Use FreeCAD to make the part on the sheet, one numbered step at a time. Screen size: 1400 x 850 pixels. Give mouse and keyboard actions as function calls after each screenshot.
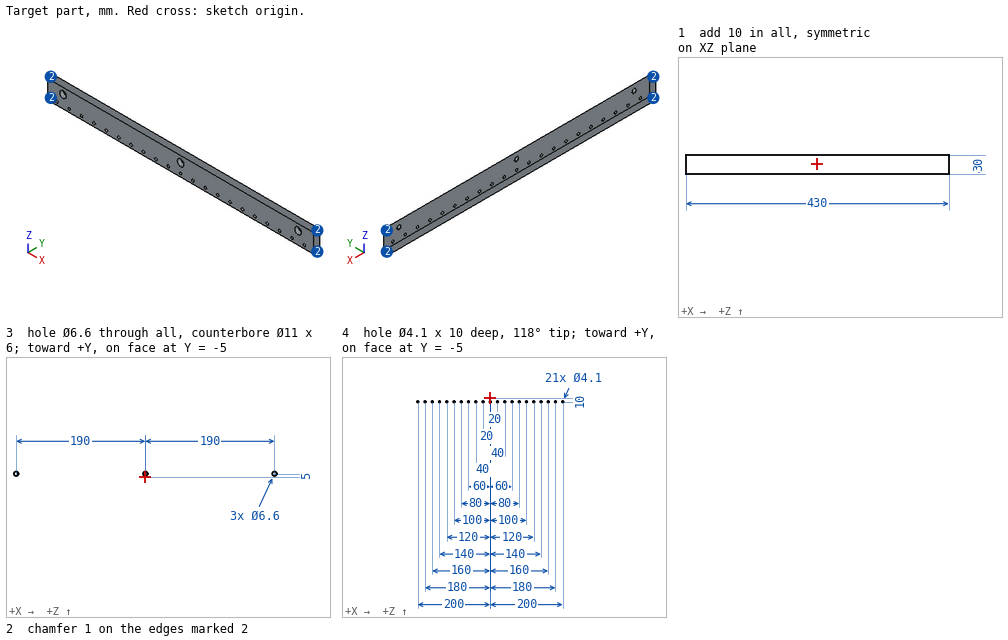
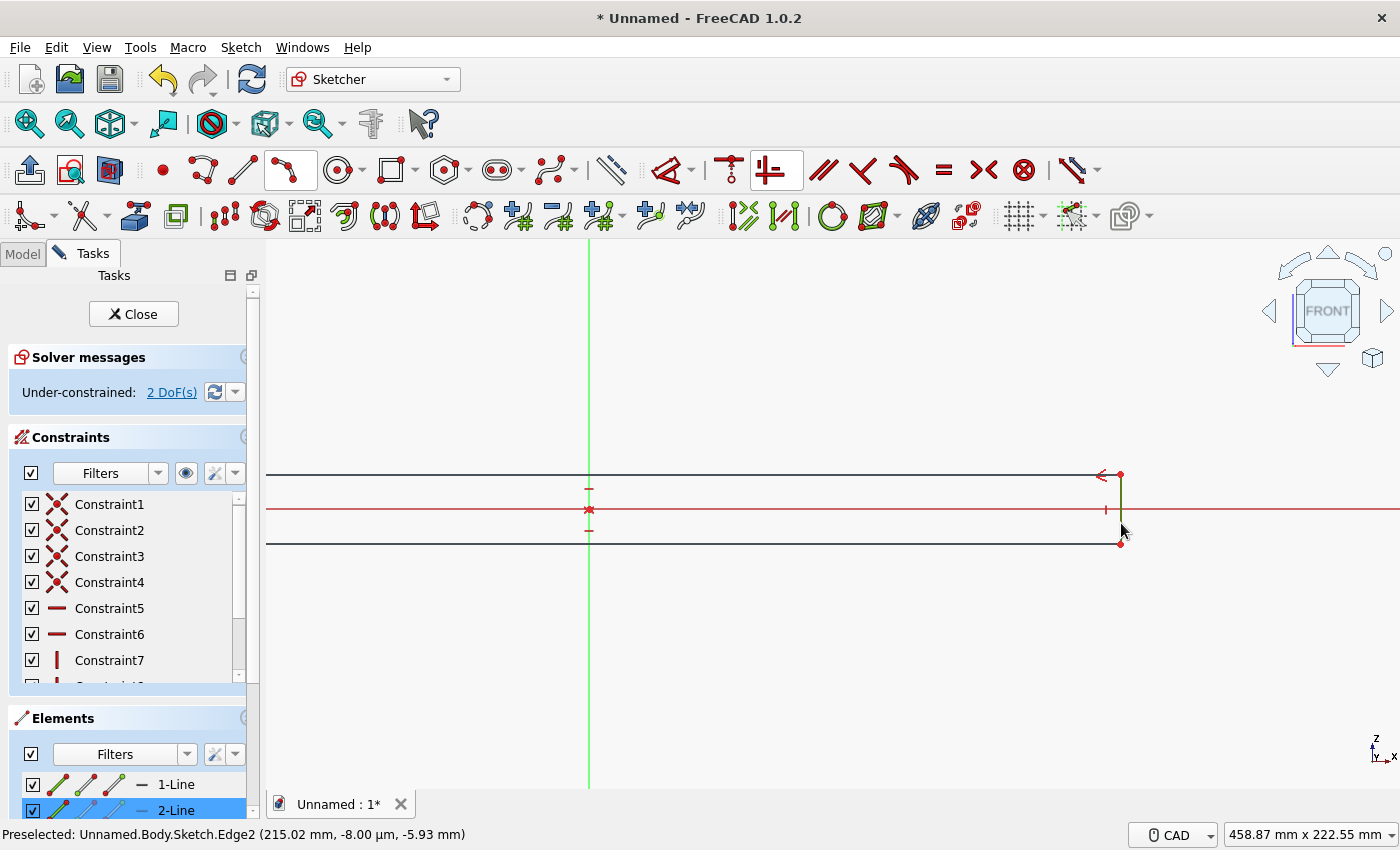
click(694, 170)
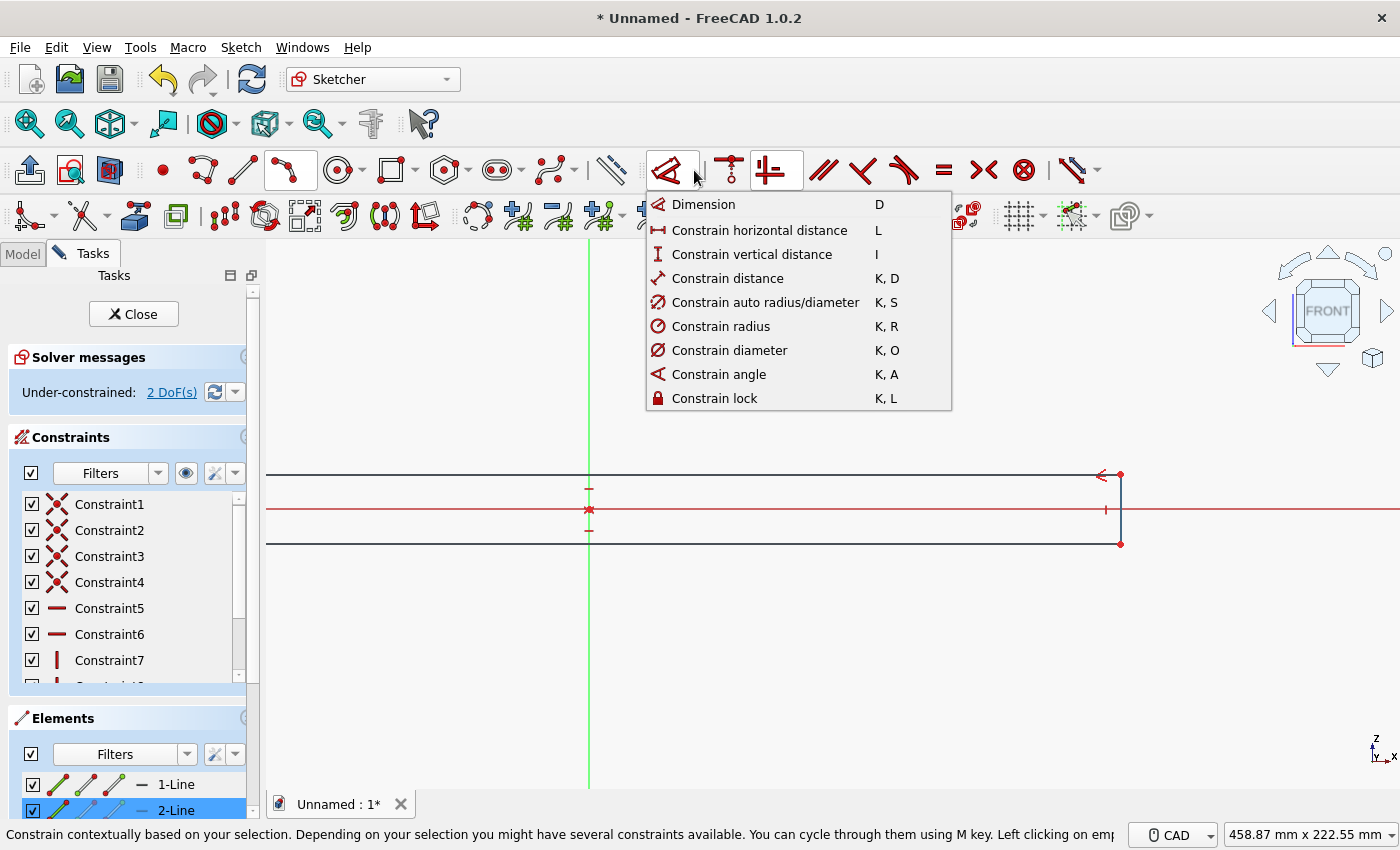
click(799, 254)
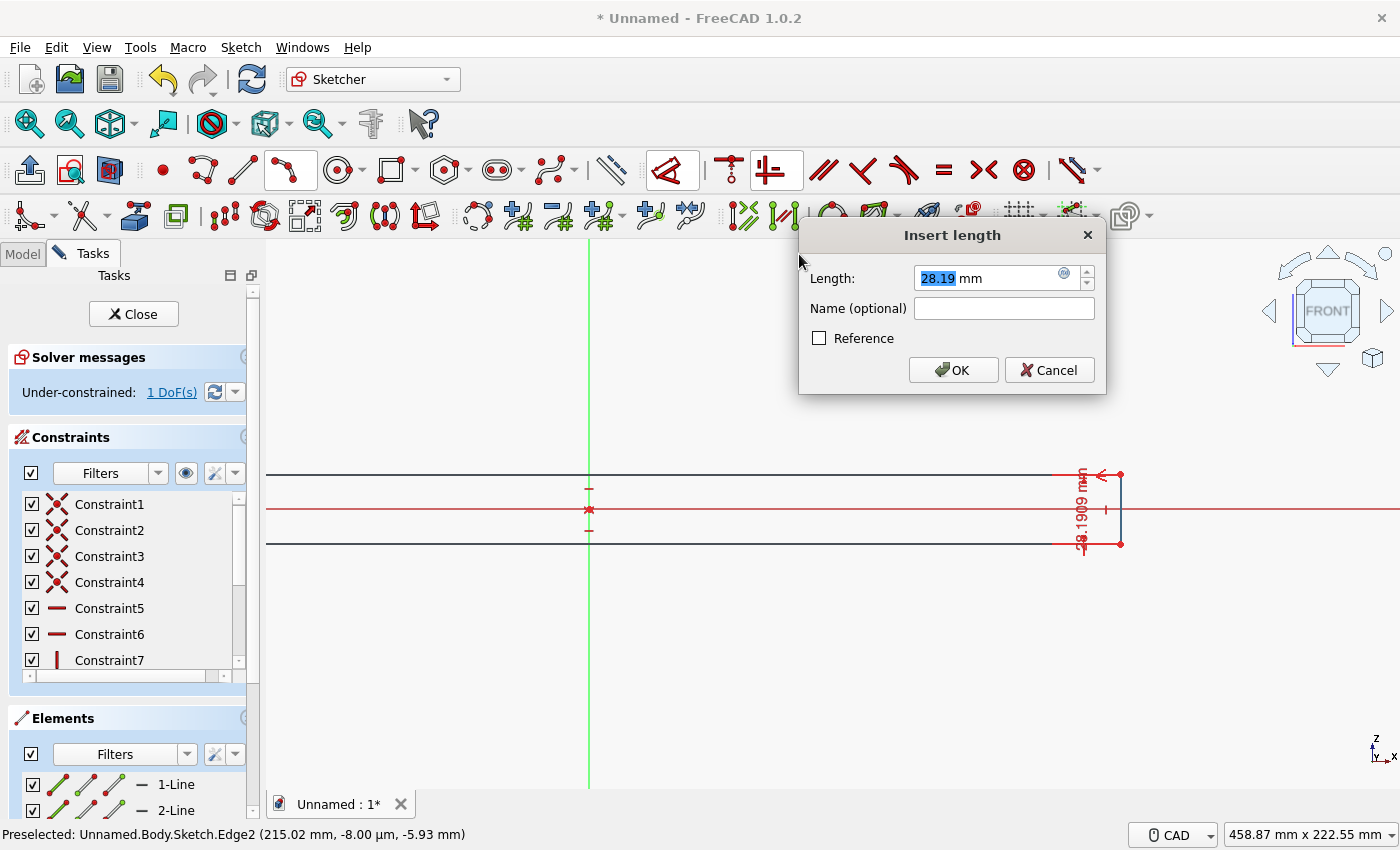
text(30)
key(Return)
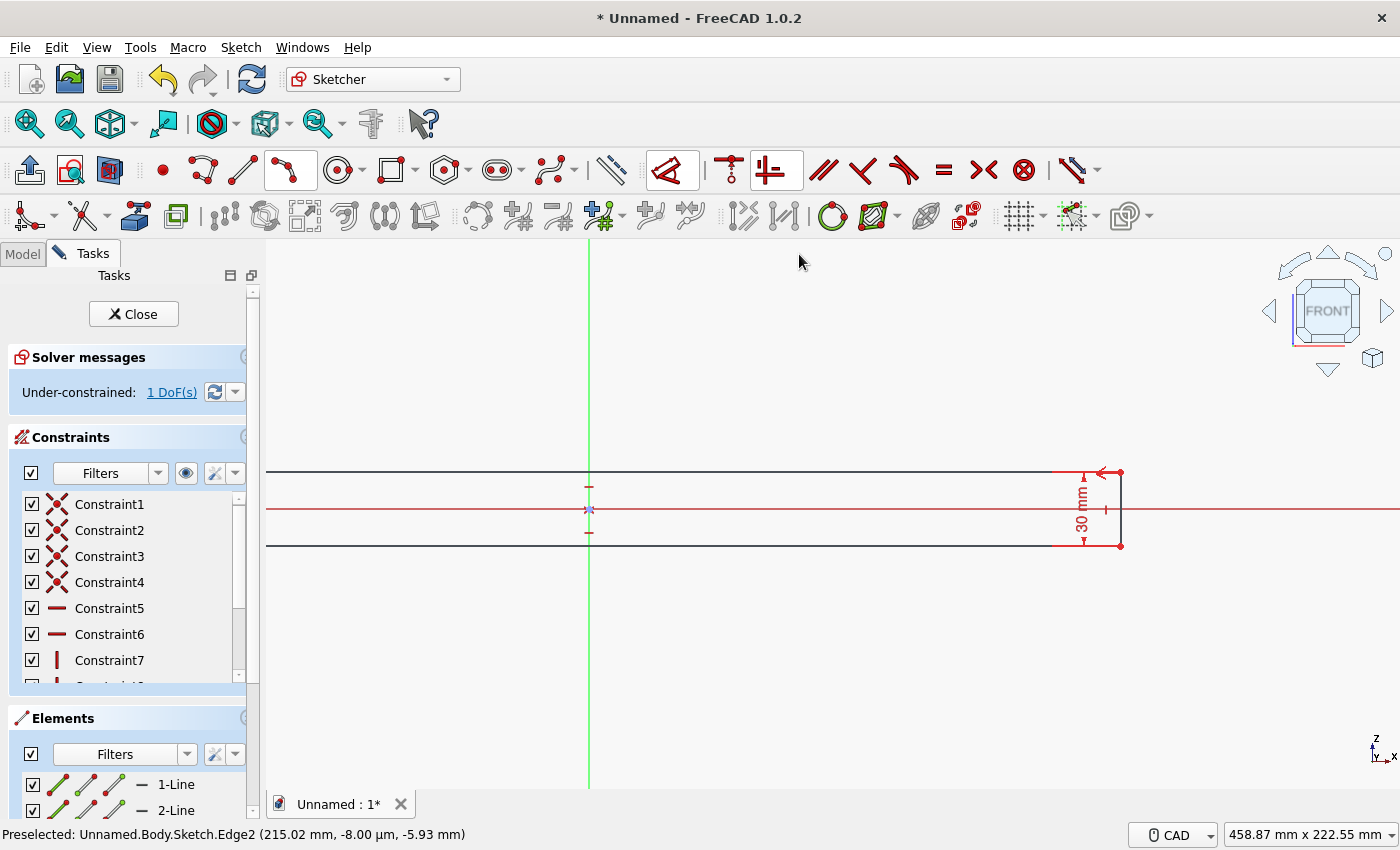
click(377, 546)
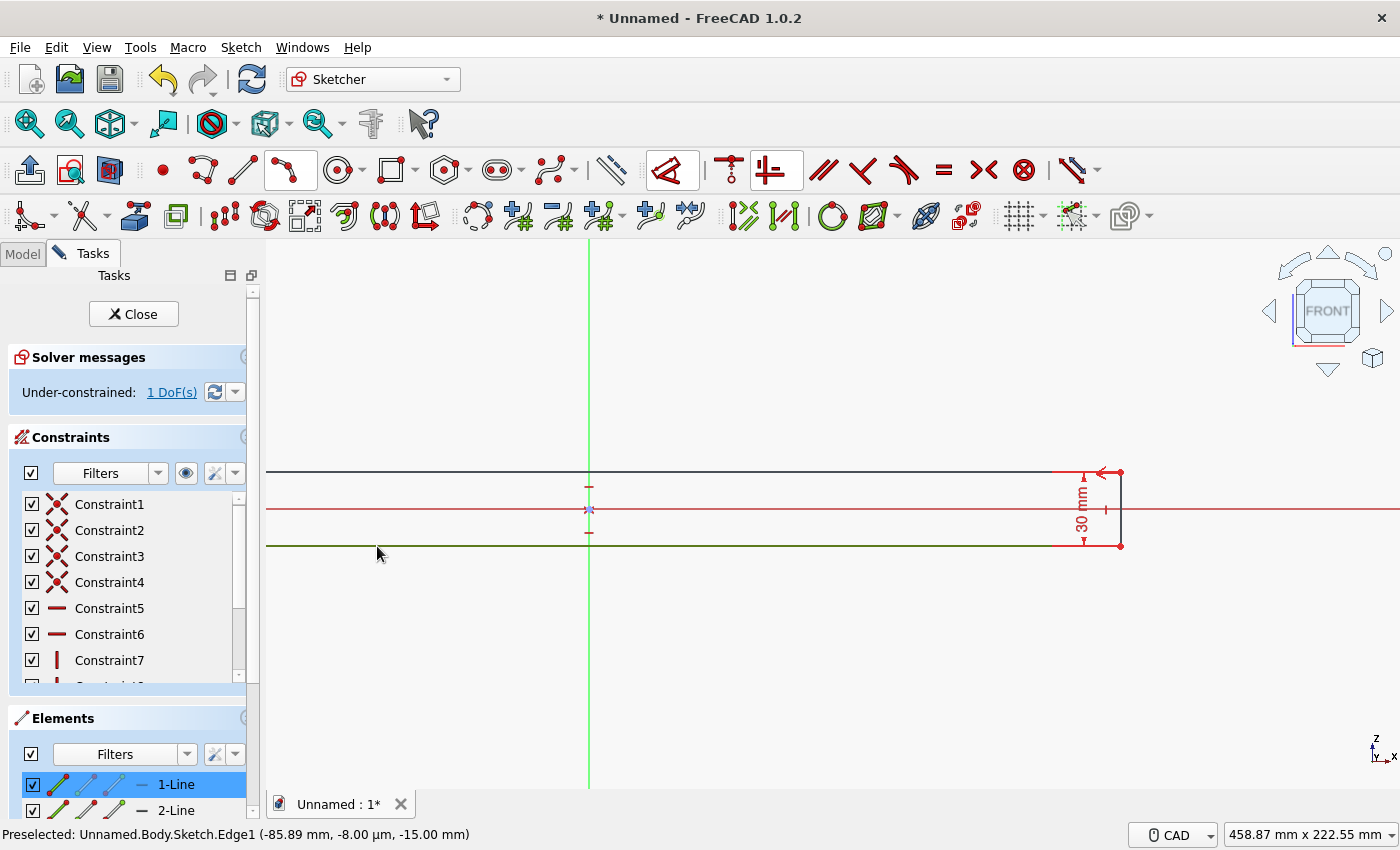
click(694, 170)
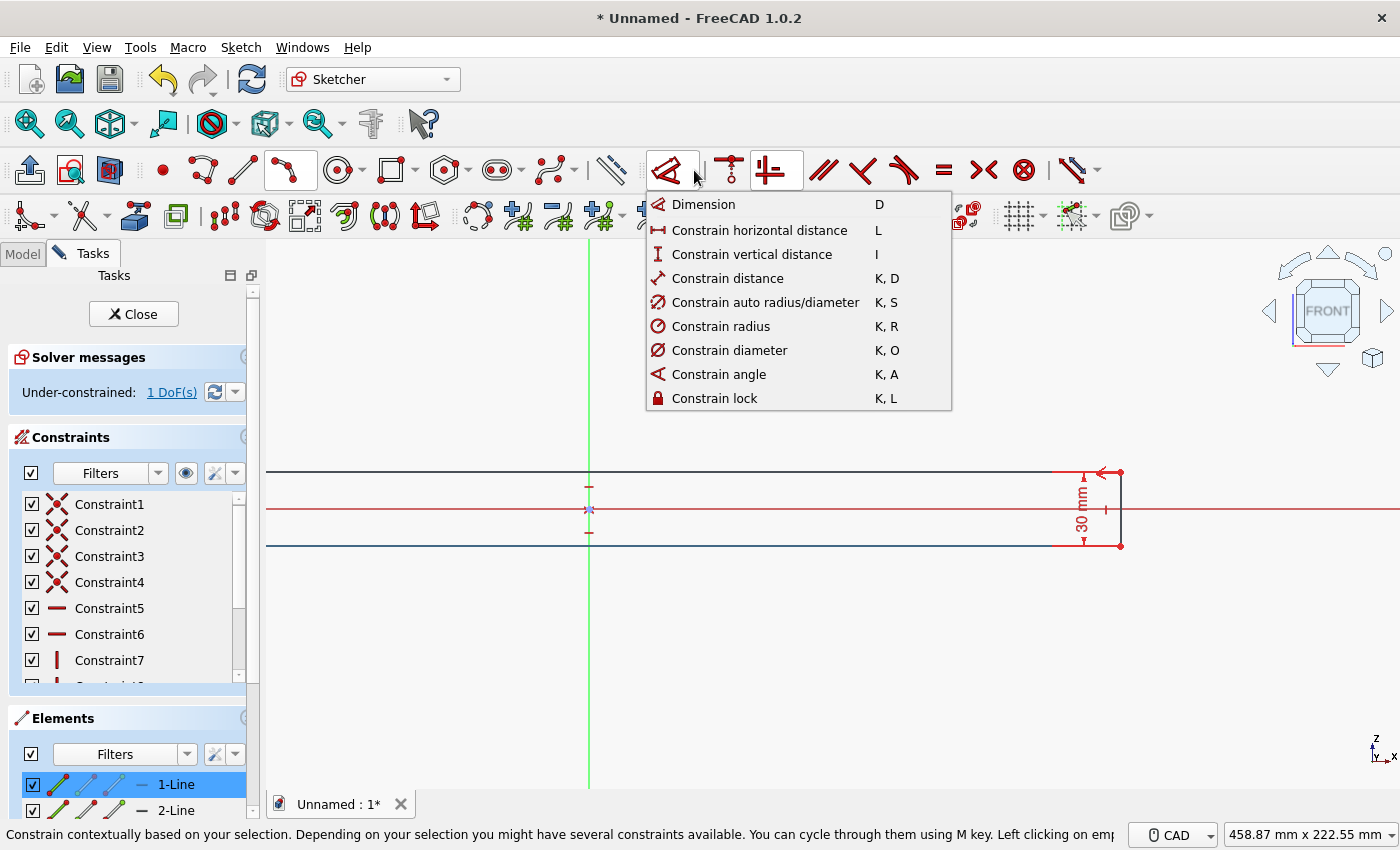
click(799, 230)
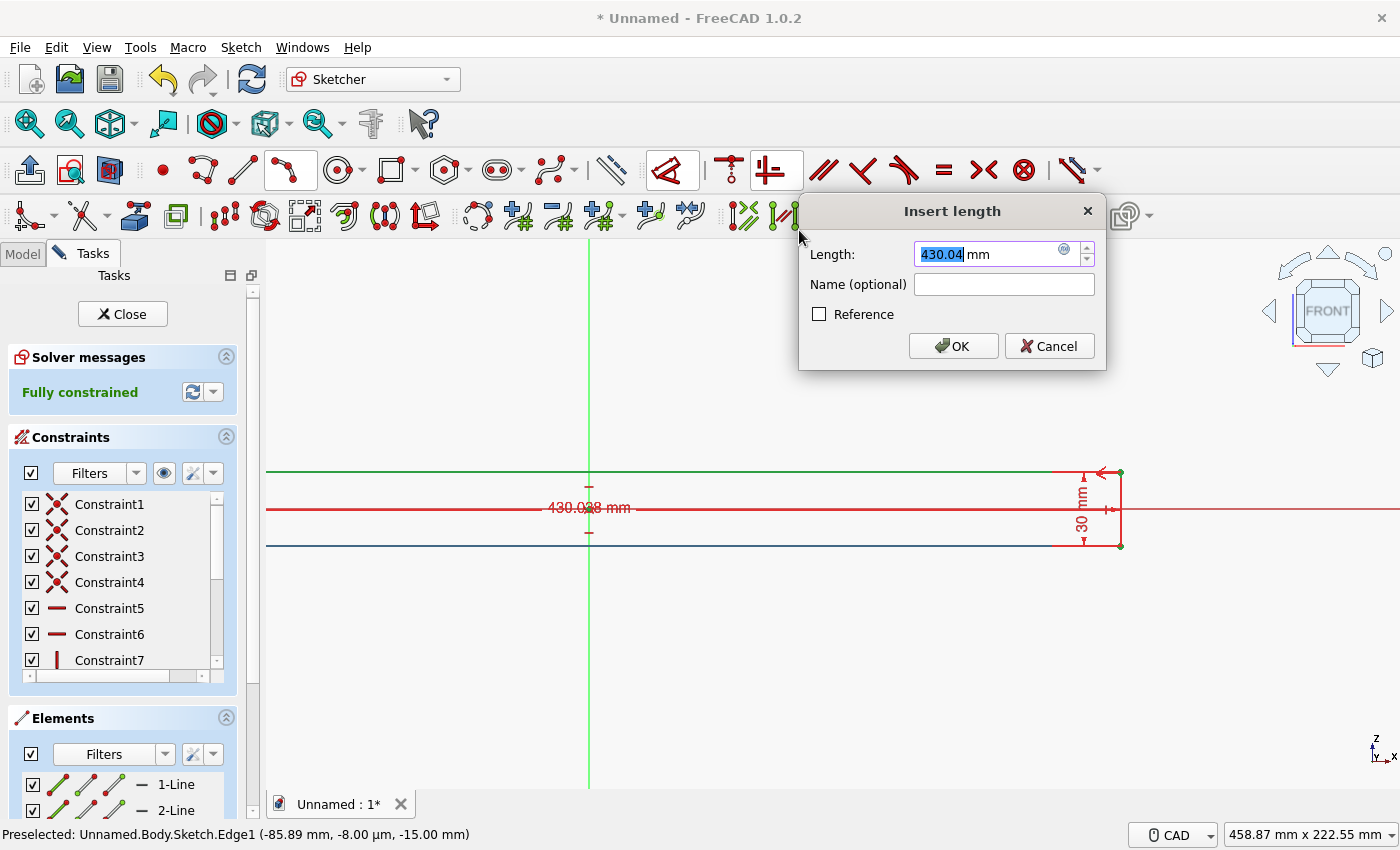
text(430)
key(Return)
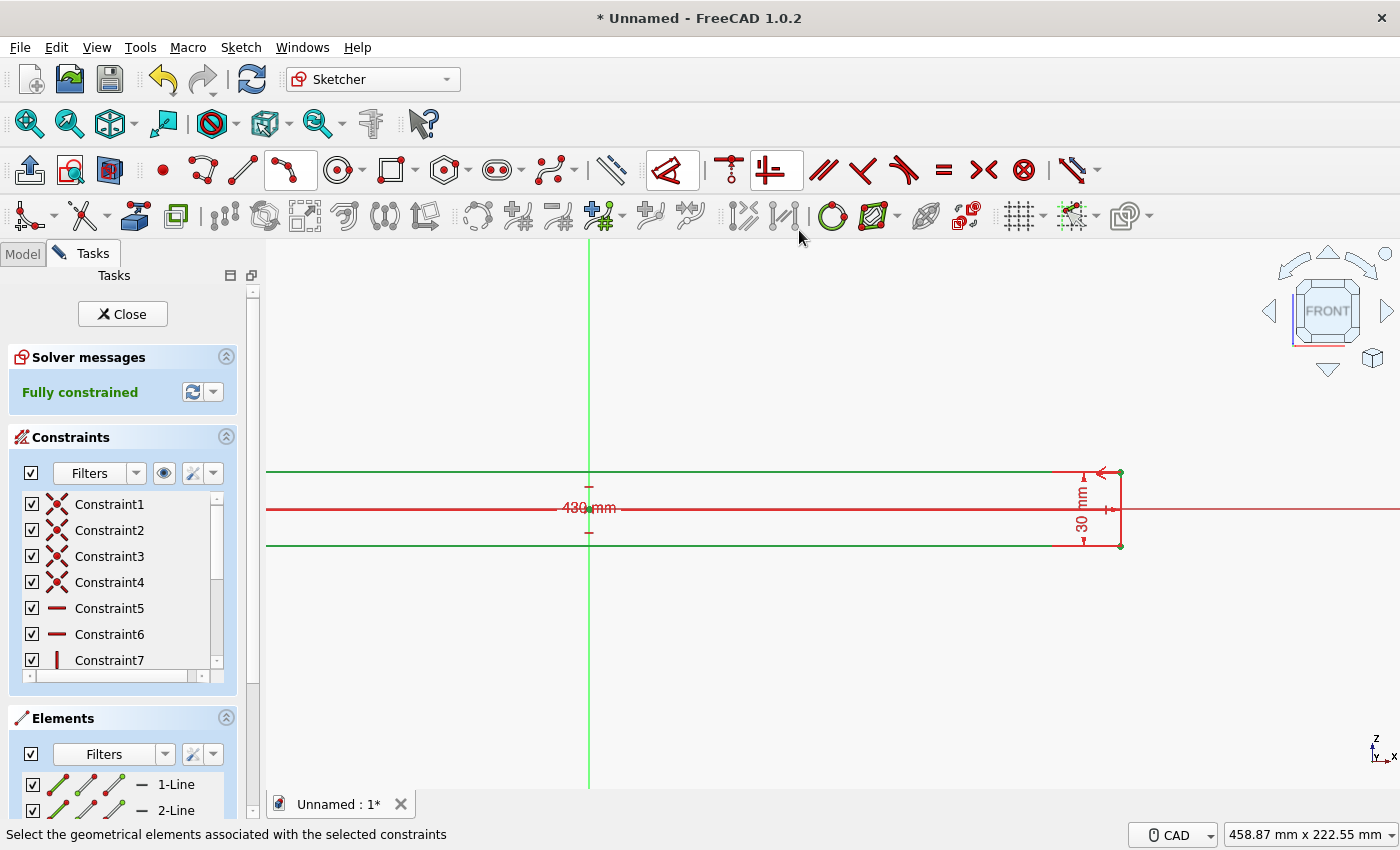
click(123, 314)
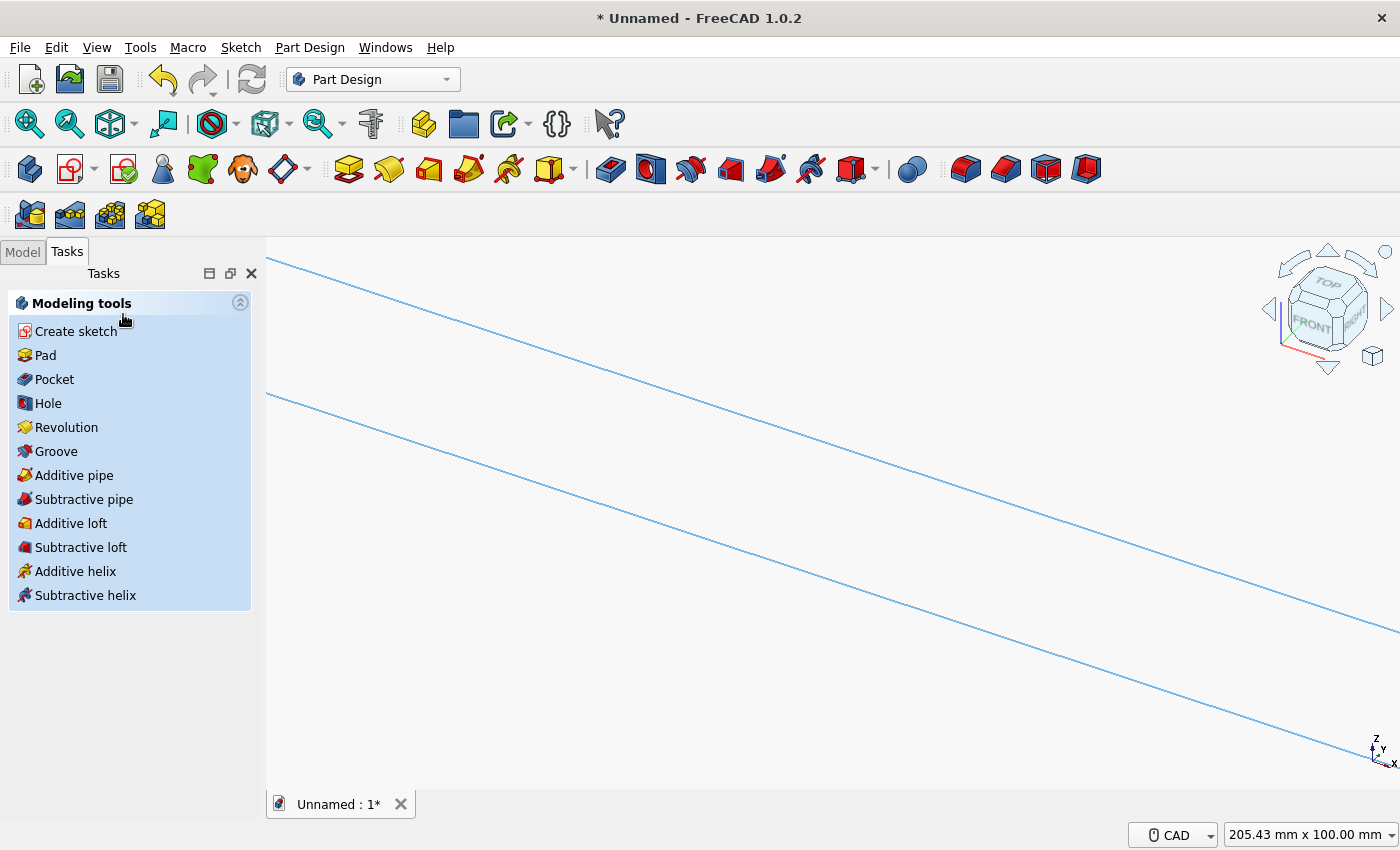
click(350, 170)